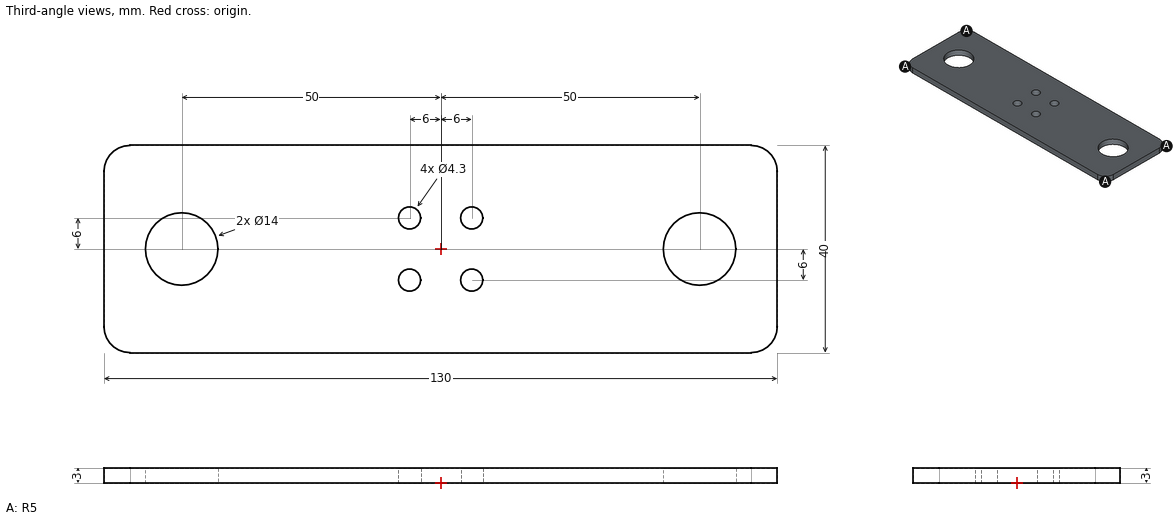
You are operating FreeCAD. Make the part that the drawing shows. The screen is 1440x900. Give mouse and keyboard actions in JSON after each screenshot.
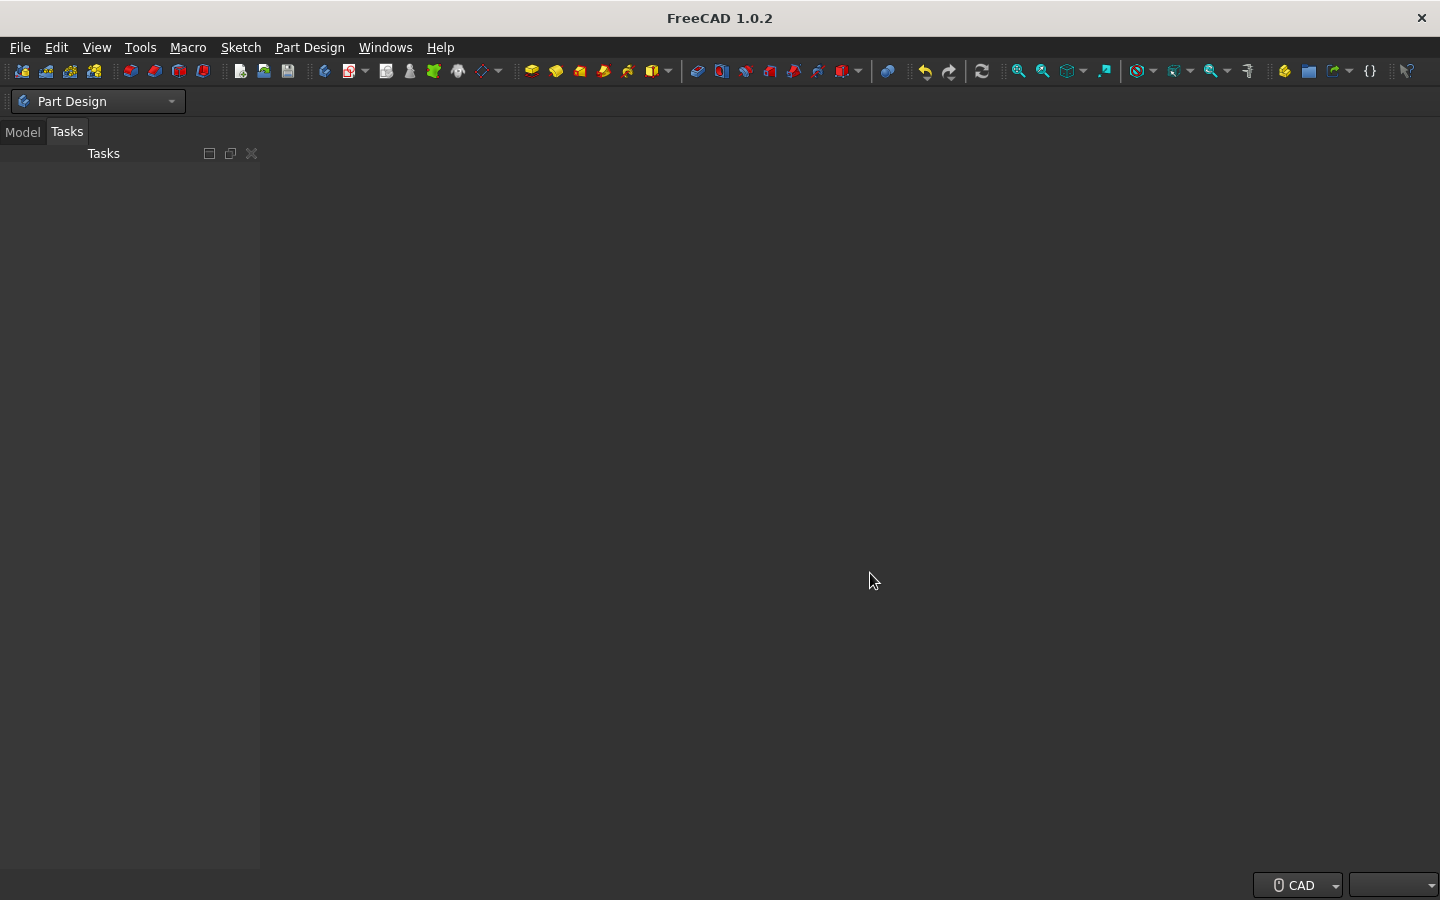
{"action": "left_click", "coordinate": [240, 72]}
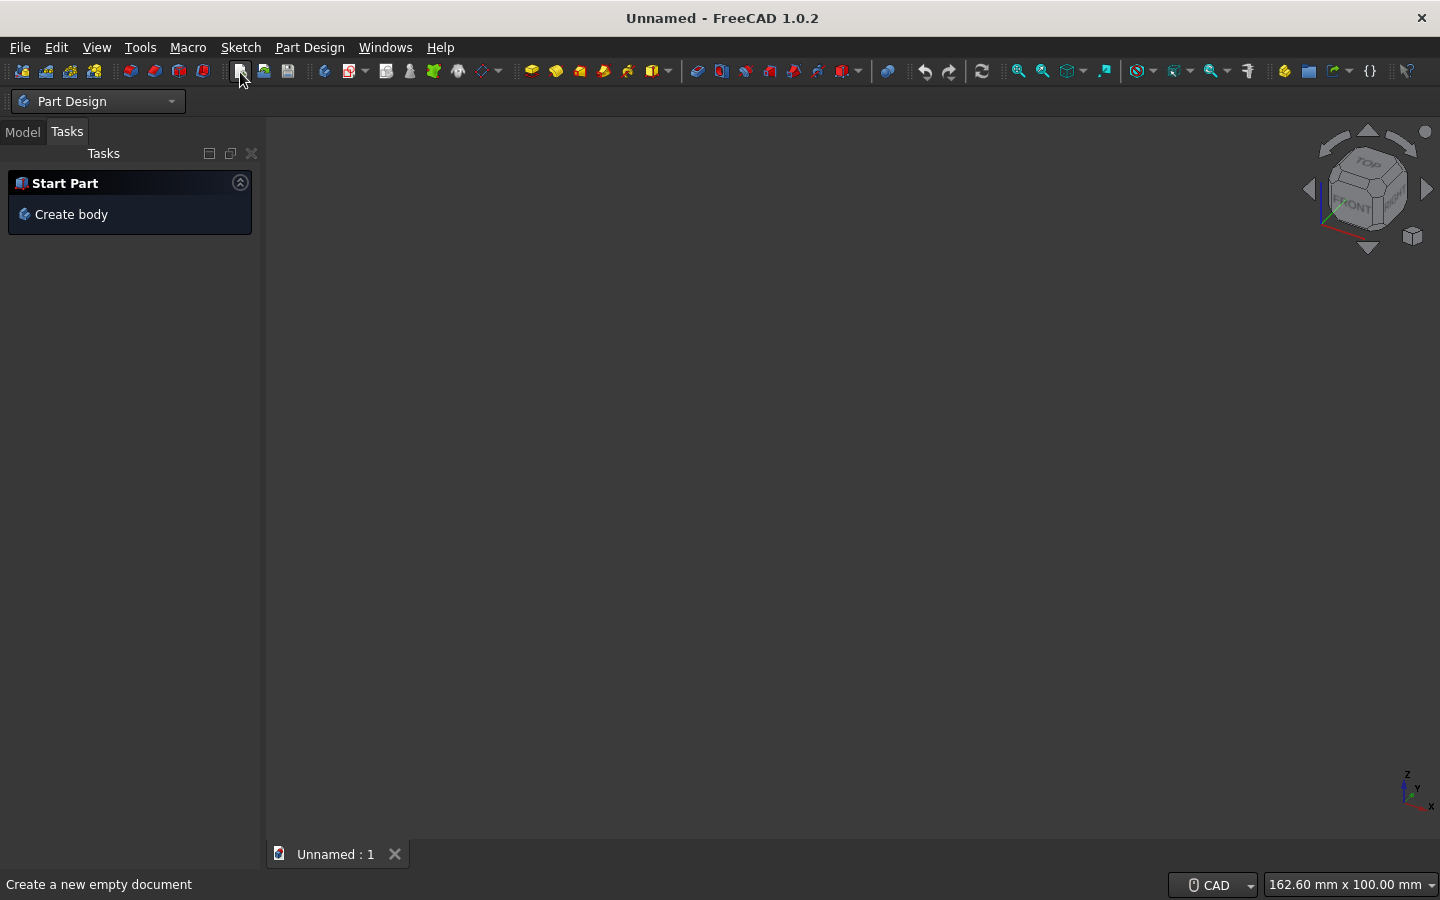
{"action": "left_click", "coordinate": [350, 72]}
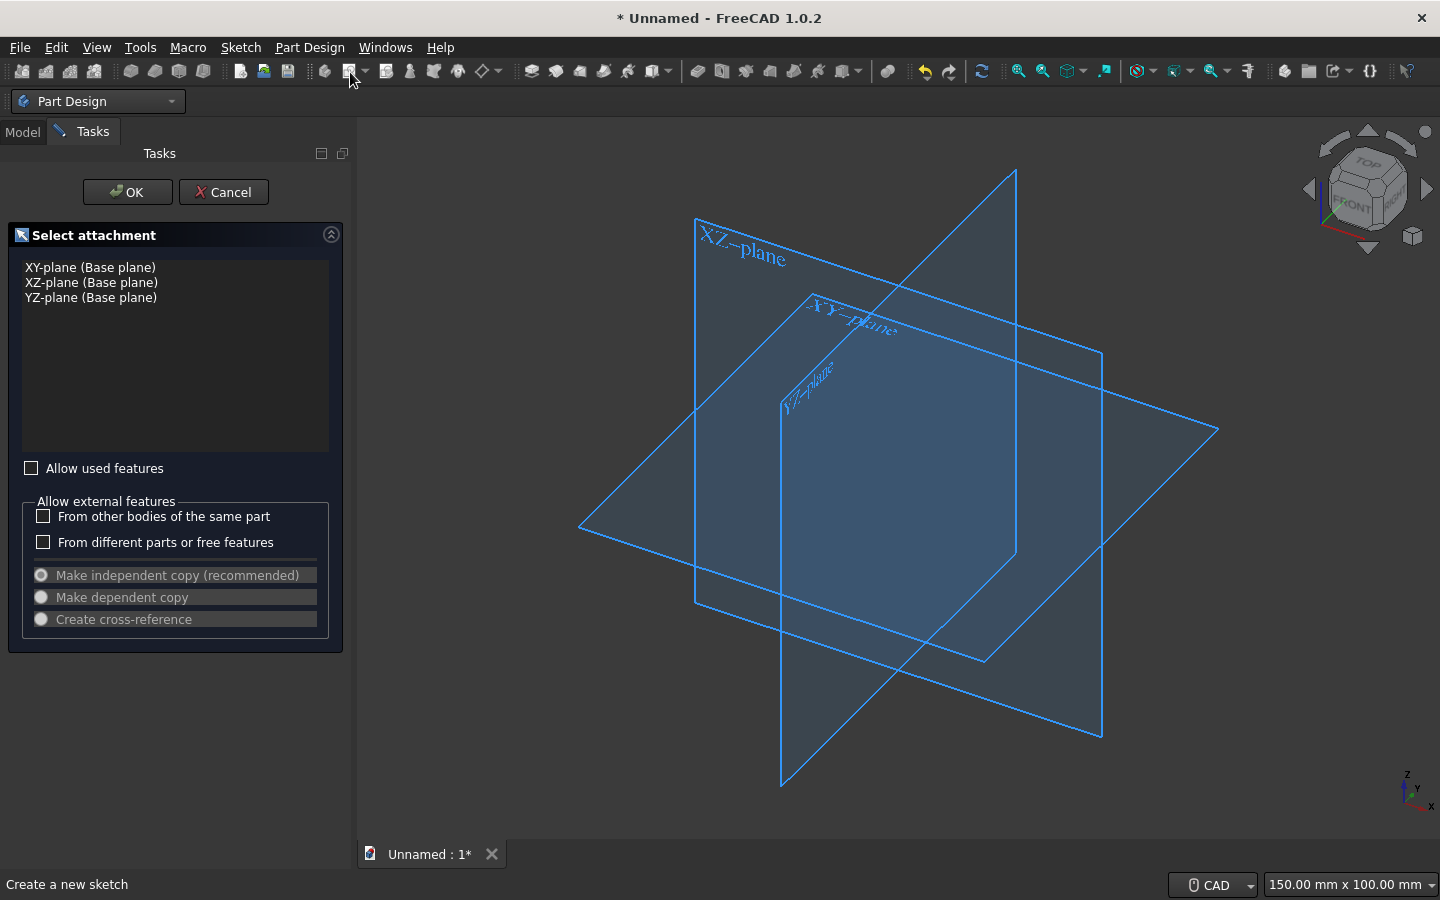
{"action": "left_click", "coordinate": [82, 268]}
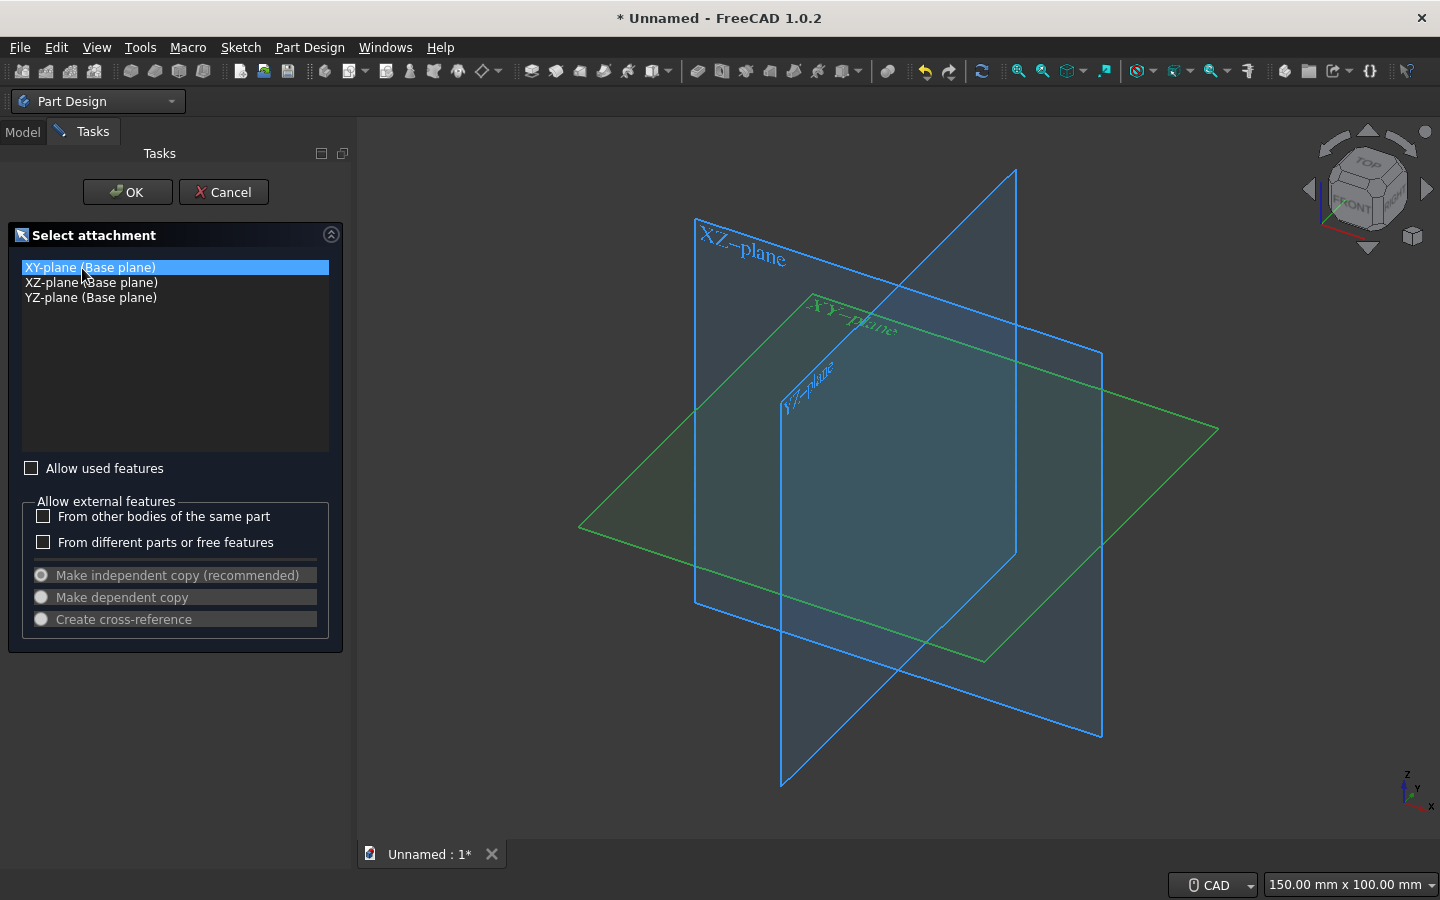
{"action": "left_click", "coordinate": [128, 192]}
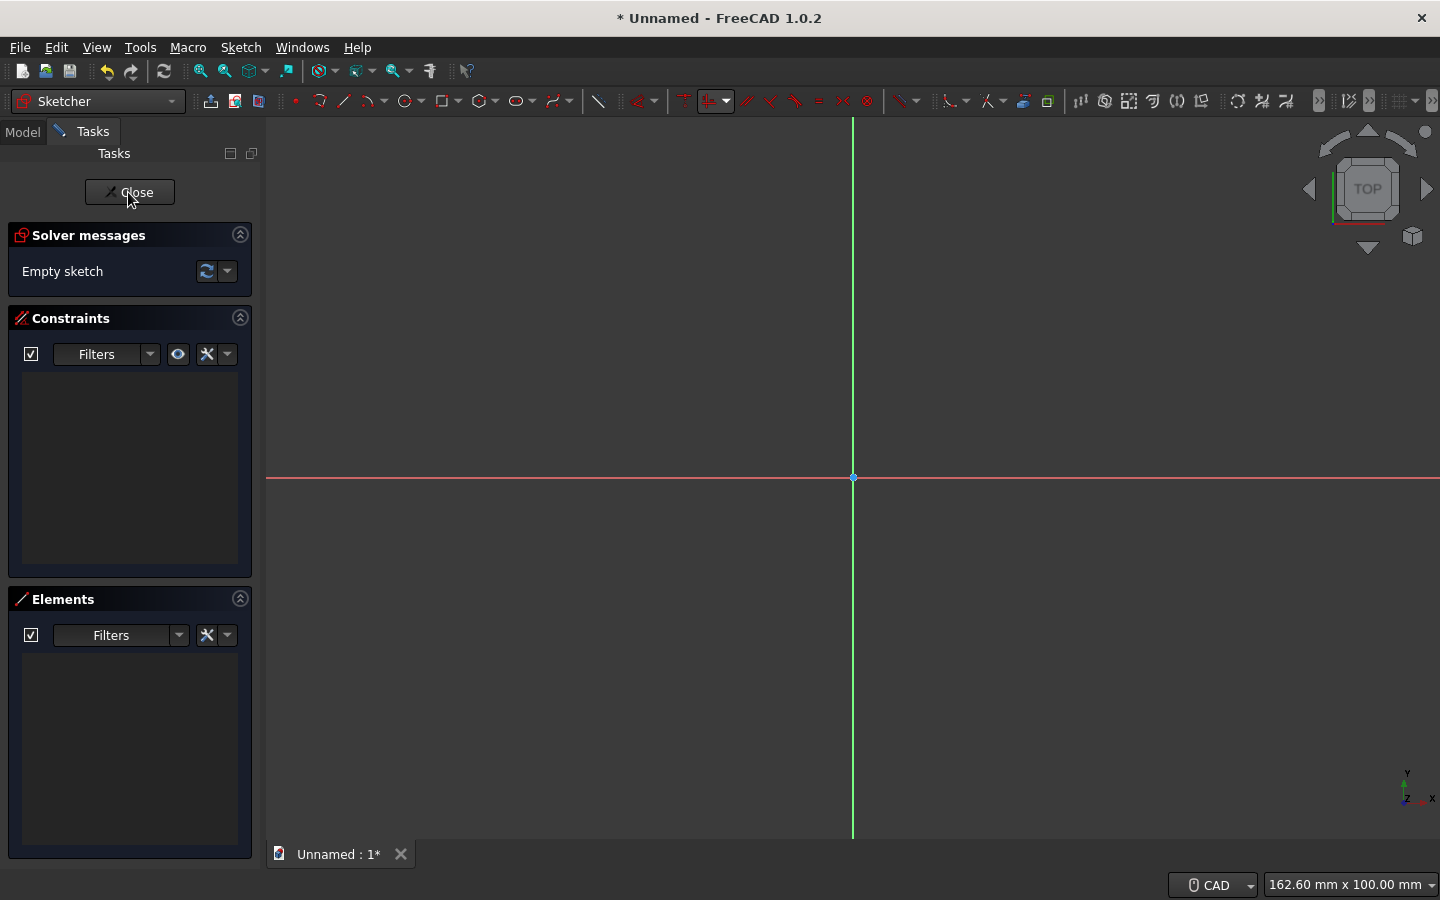
{"action": "scroll", "coordinate": [645, 478], "scroll_direction": "down", "scroll_amount": 2}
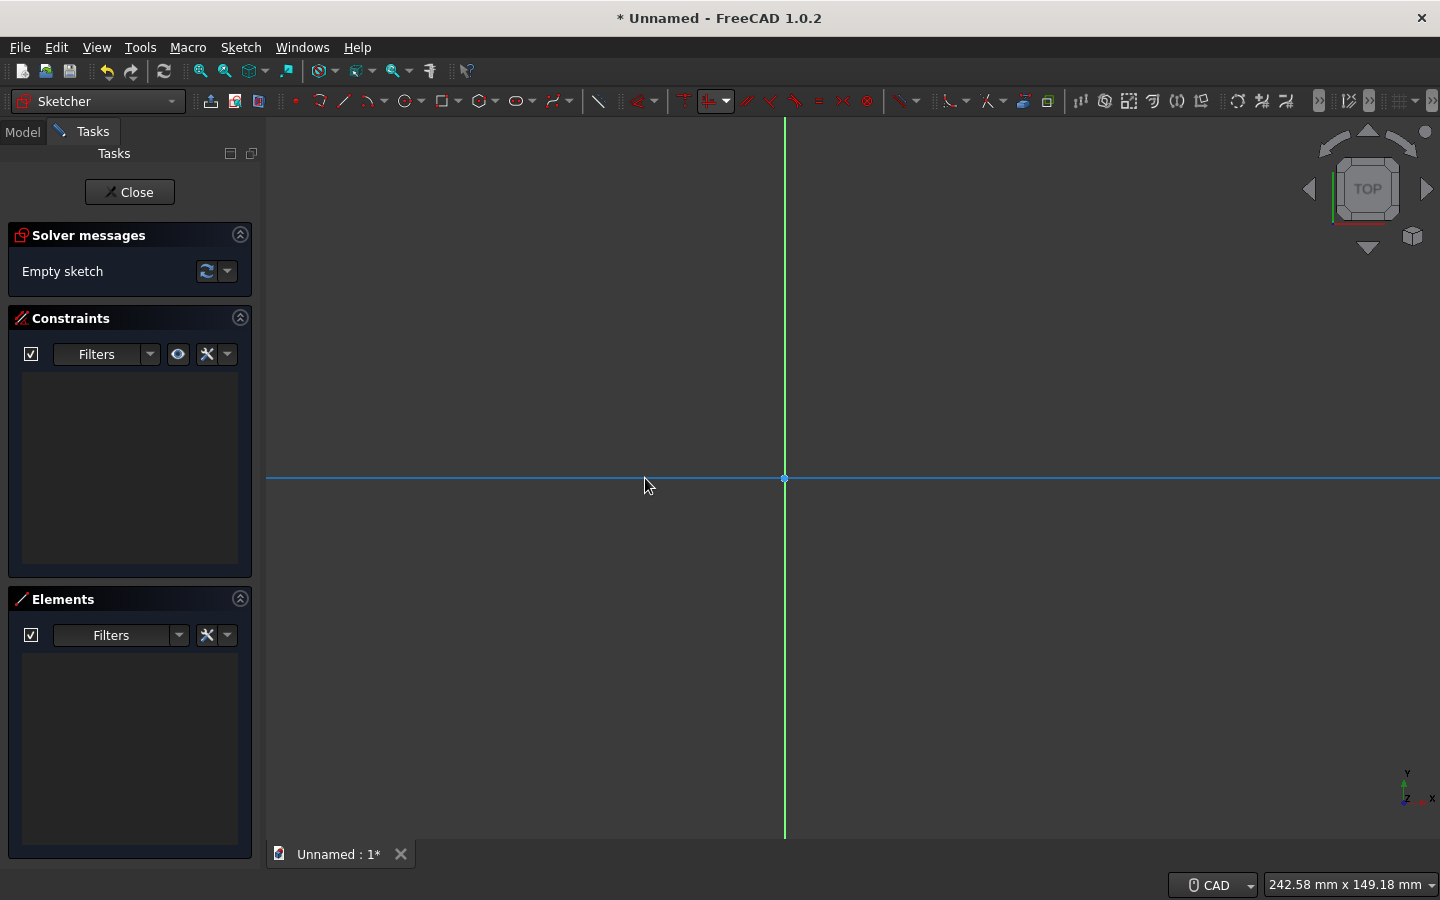
{"action": "key", "text": "g v"}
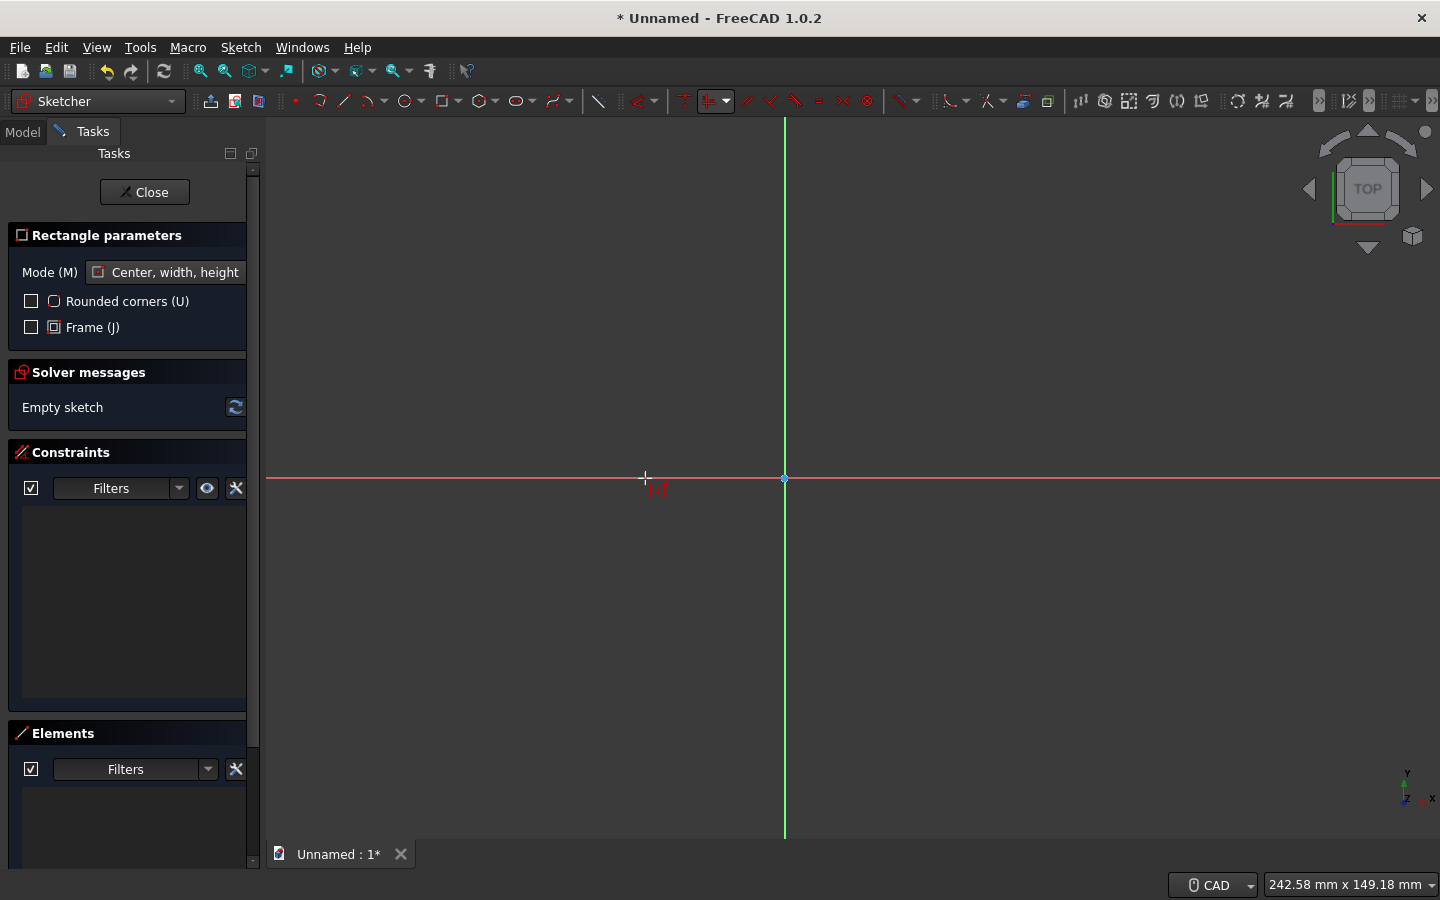
{"action": "left_click", "coordinate": [785, 478]}
{"action": "left_click", "coordinate": [1099, 381]}
{"action": "key", "text": "Escape"}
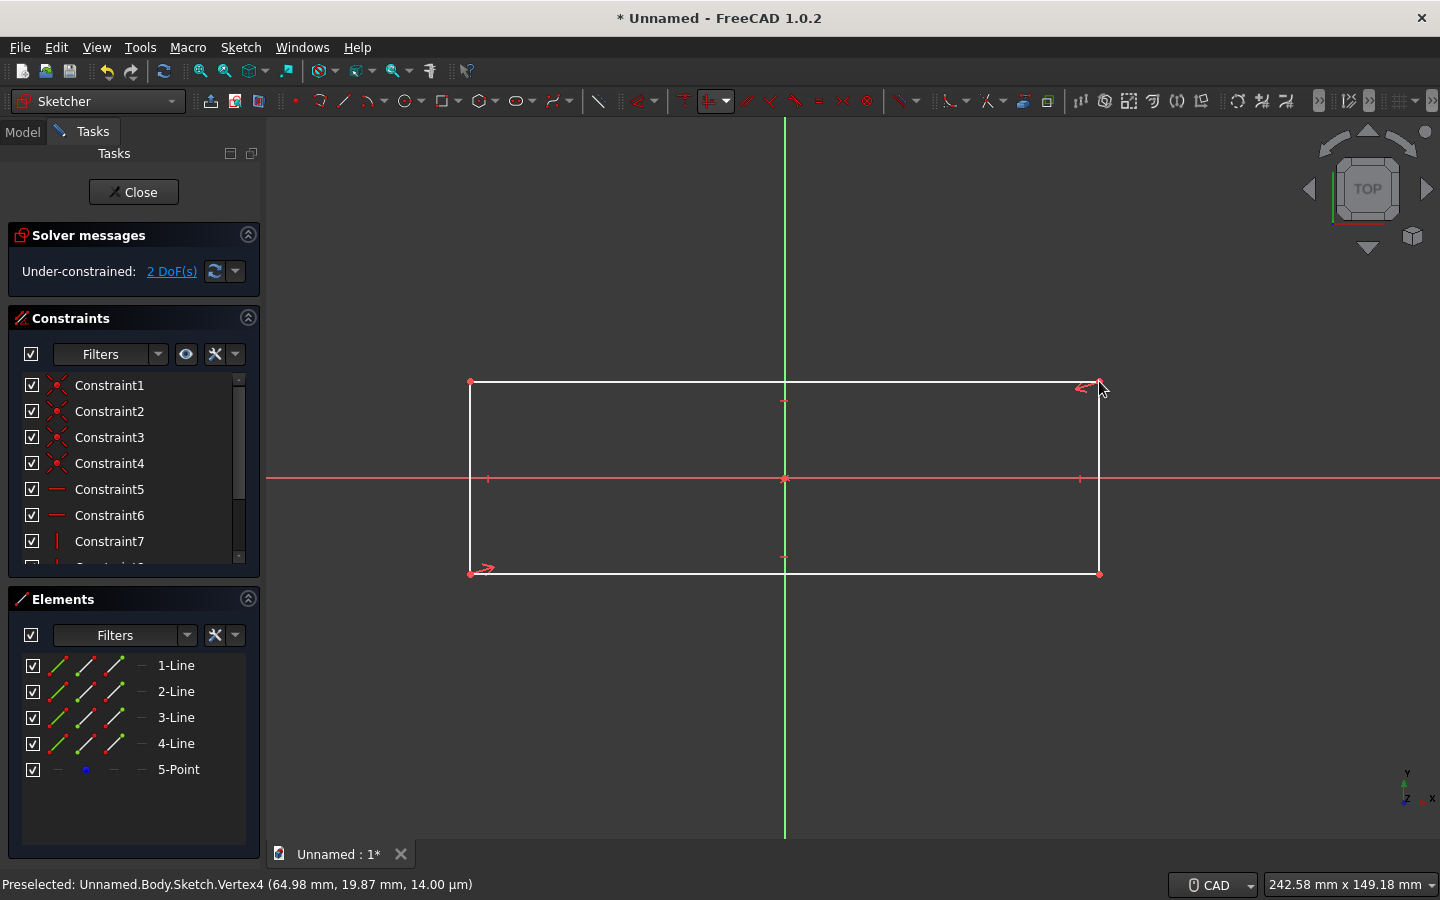
{"action": "left_click", "coordinate": [1099, 517]}